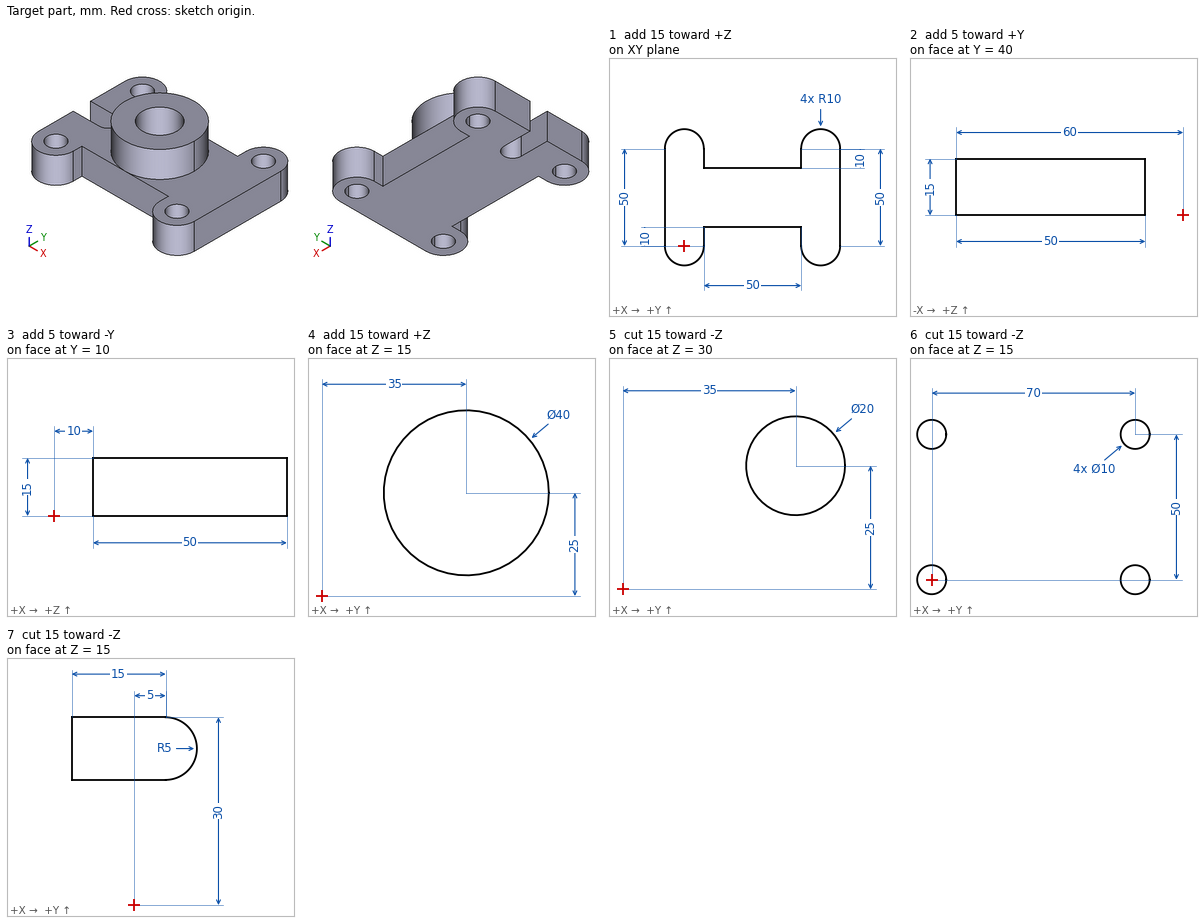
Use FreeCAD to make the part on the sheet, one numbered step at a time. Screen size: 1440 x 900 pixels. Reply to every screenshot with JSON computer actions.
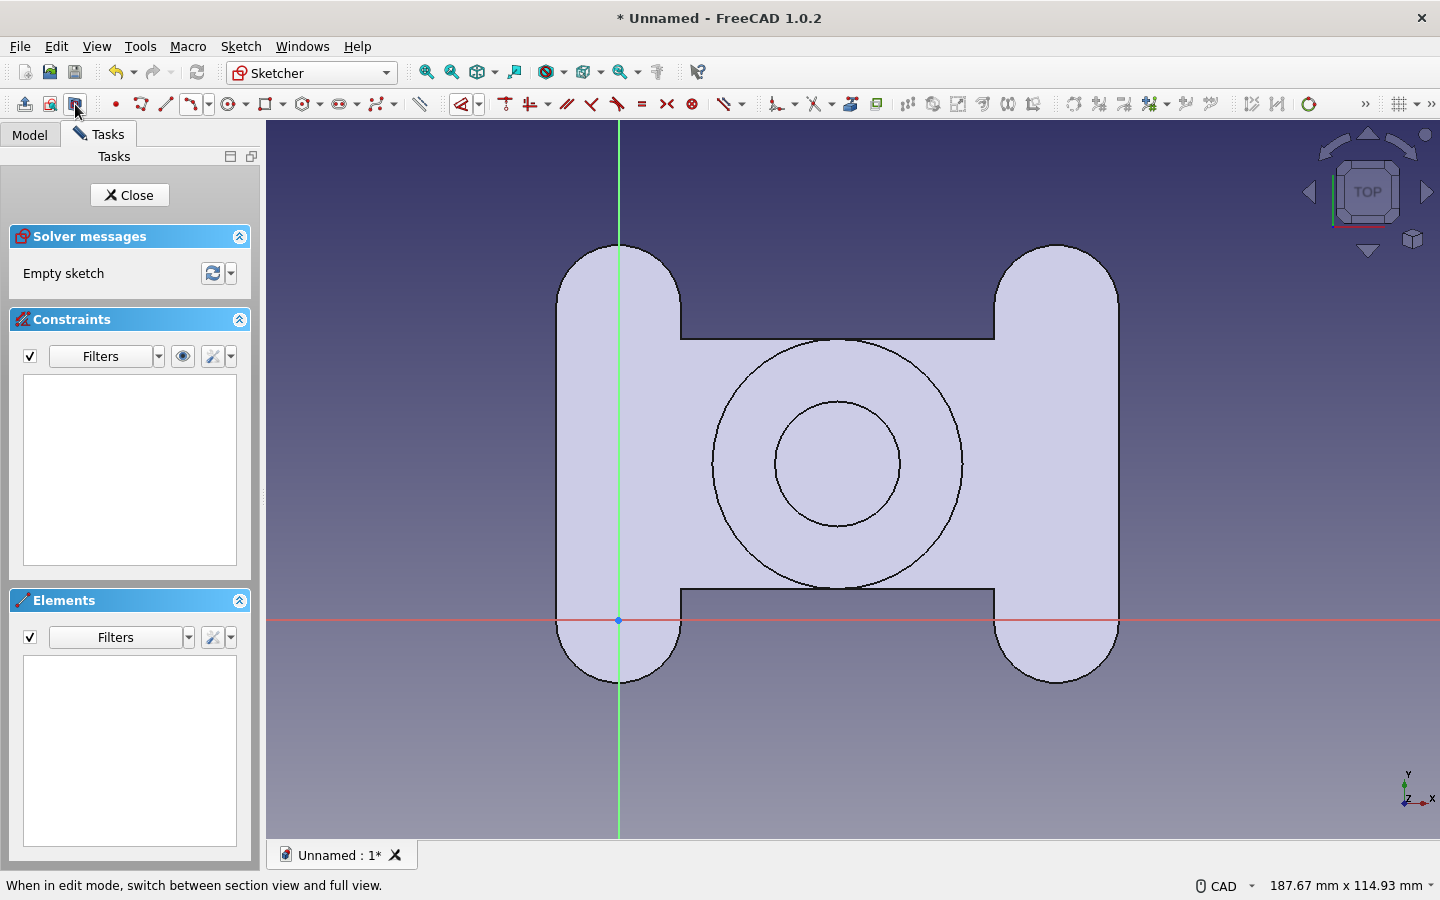
{"action": "left_click", "coordinate": [228, 104]}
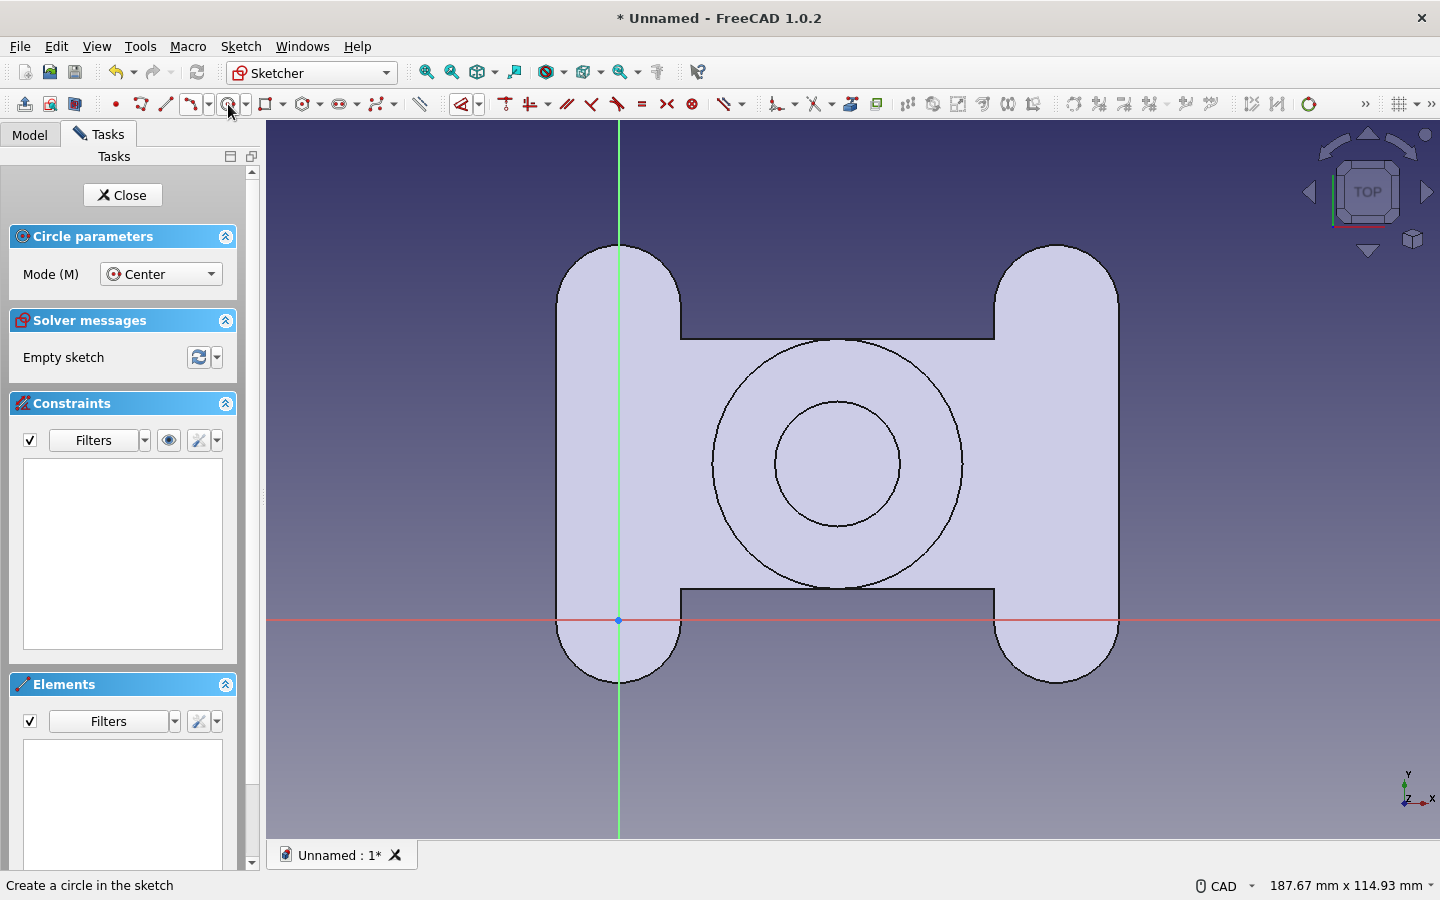
{"action": "left_click", "coordinate": [1056, 308]}
{"action": "left_click", "coordinate": [1079, 285]}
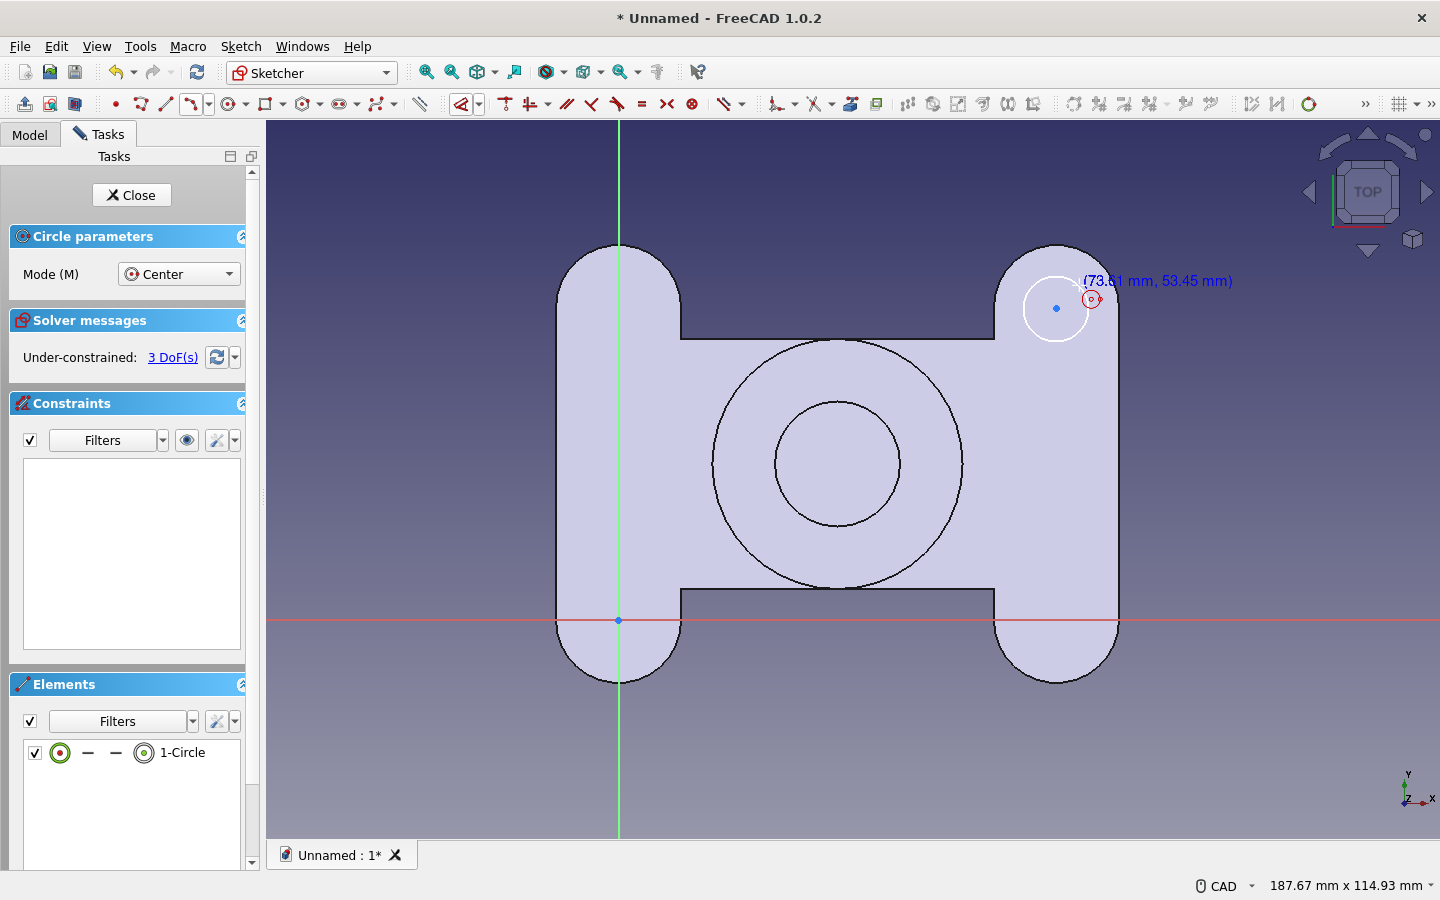
{"action": "left_click", "coordinate": [1056, 620]}
{"action": "left_click", "coordinate": [1079, 598]}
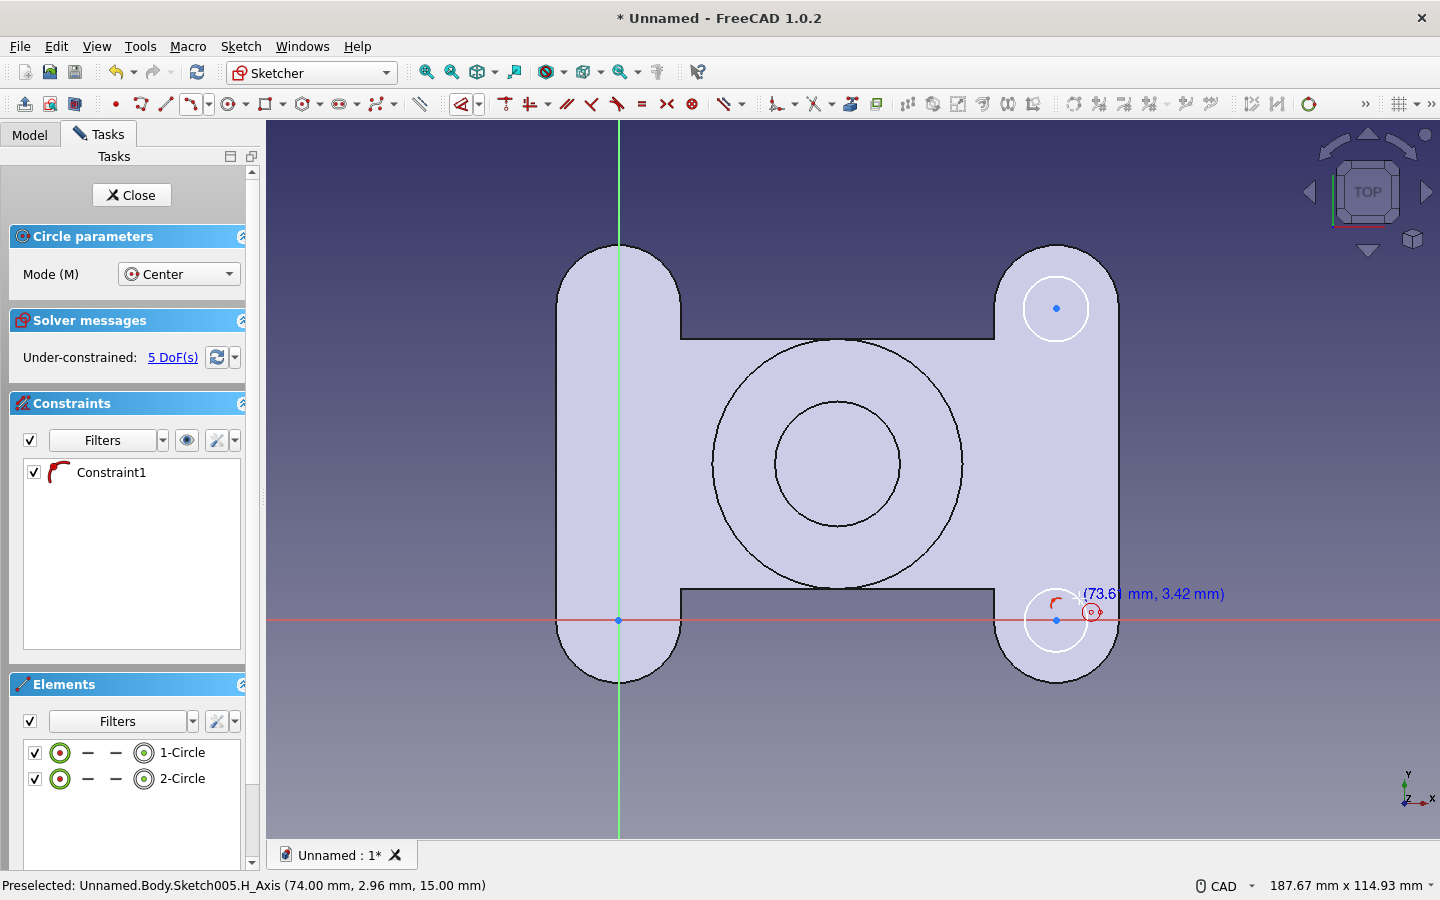
{"action": "left_click", "coordinate": [619, 620]}
{"action": "left_click", "coordinate": [641, 598]}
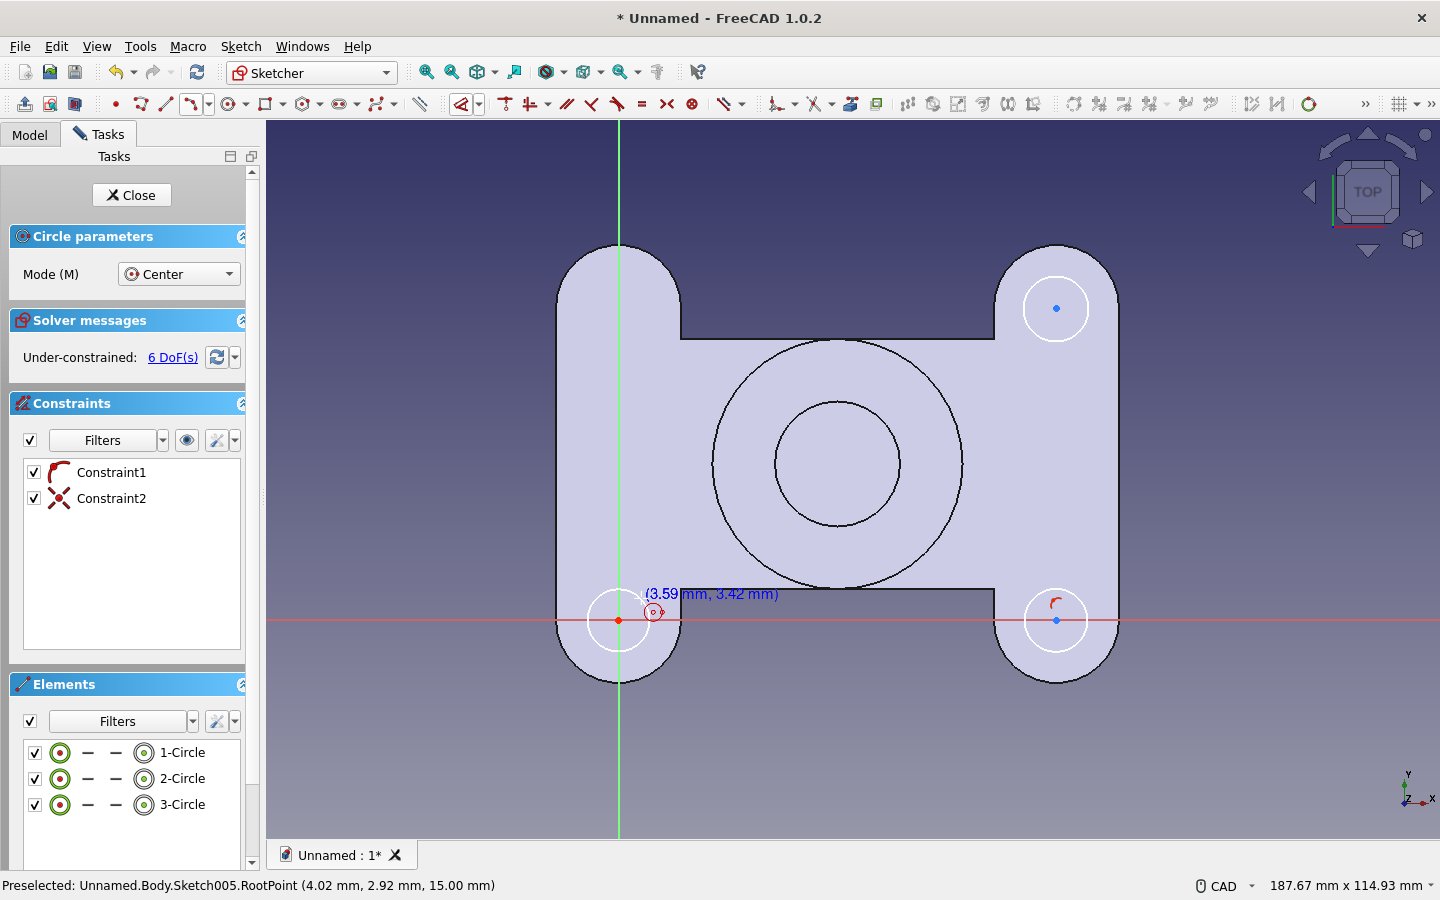
{"action": "left_click", "coordinate": [619, 308]}
{"action": "left_click", "coordinate": [641, 285]}
{"action": "key", "text": "Escape"}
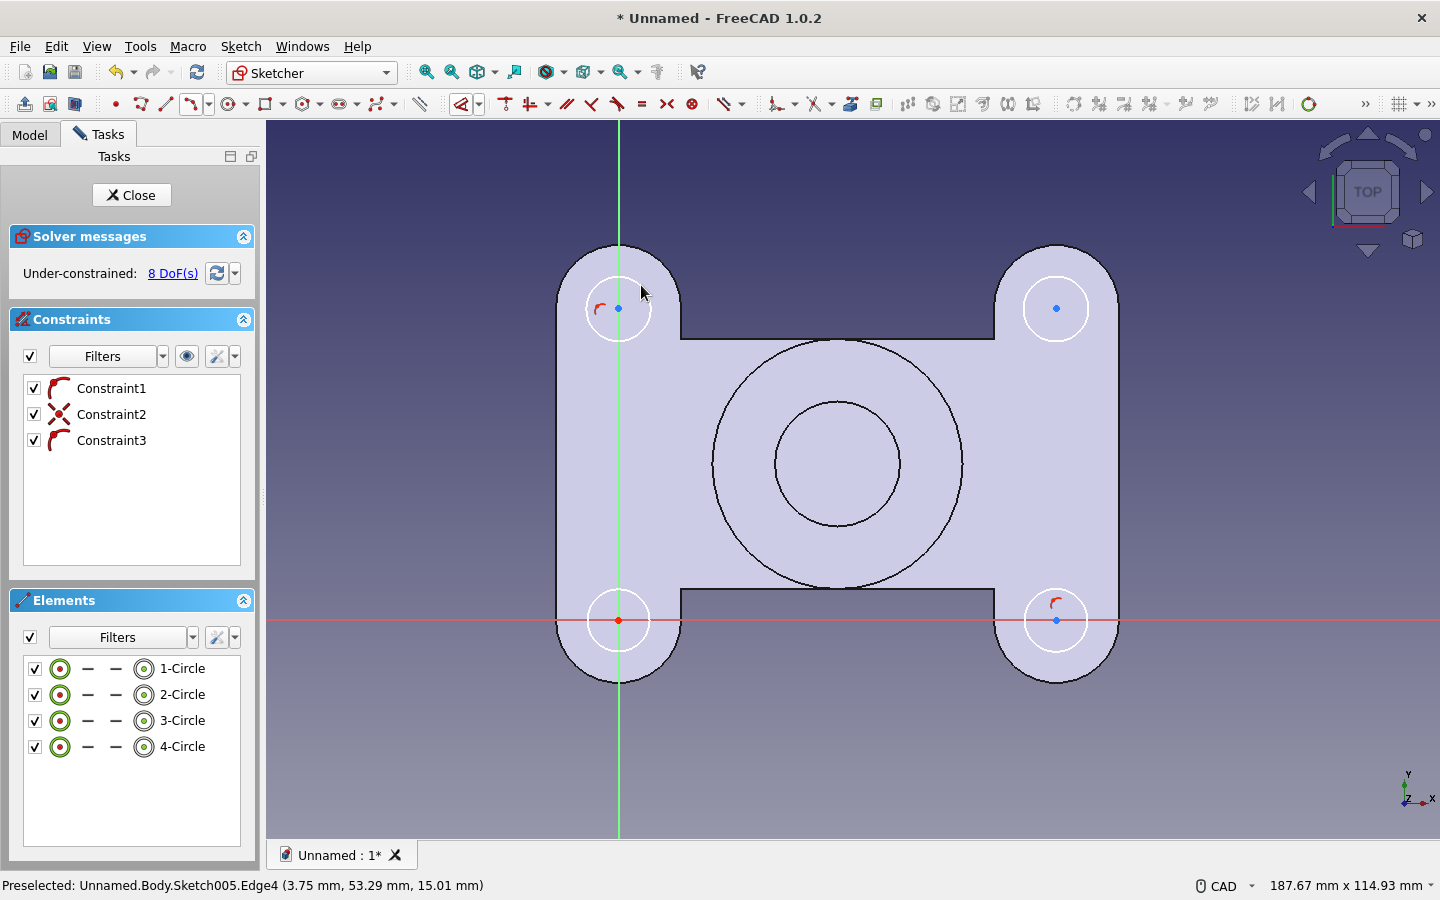
{"action": "left_click", "coordinate": [1079, 286]}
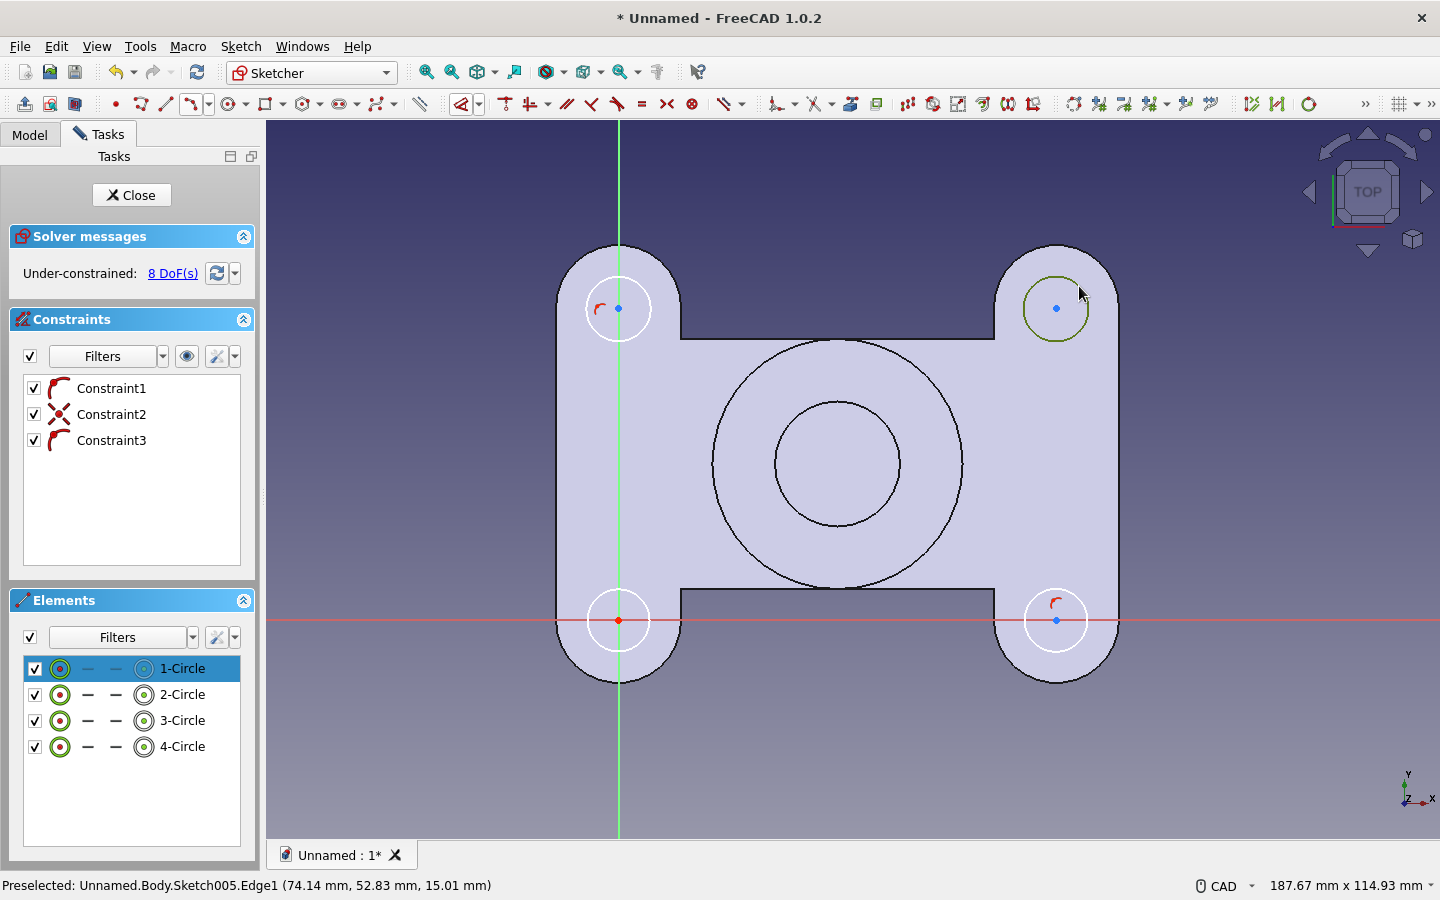
{"action": "left_click", "coordinate": [1078, 598]}